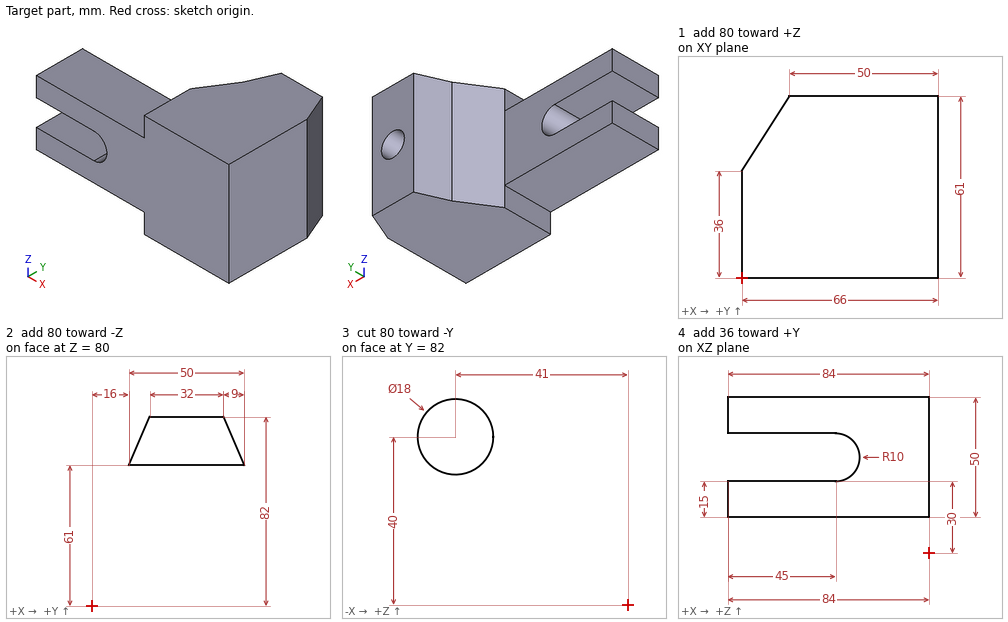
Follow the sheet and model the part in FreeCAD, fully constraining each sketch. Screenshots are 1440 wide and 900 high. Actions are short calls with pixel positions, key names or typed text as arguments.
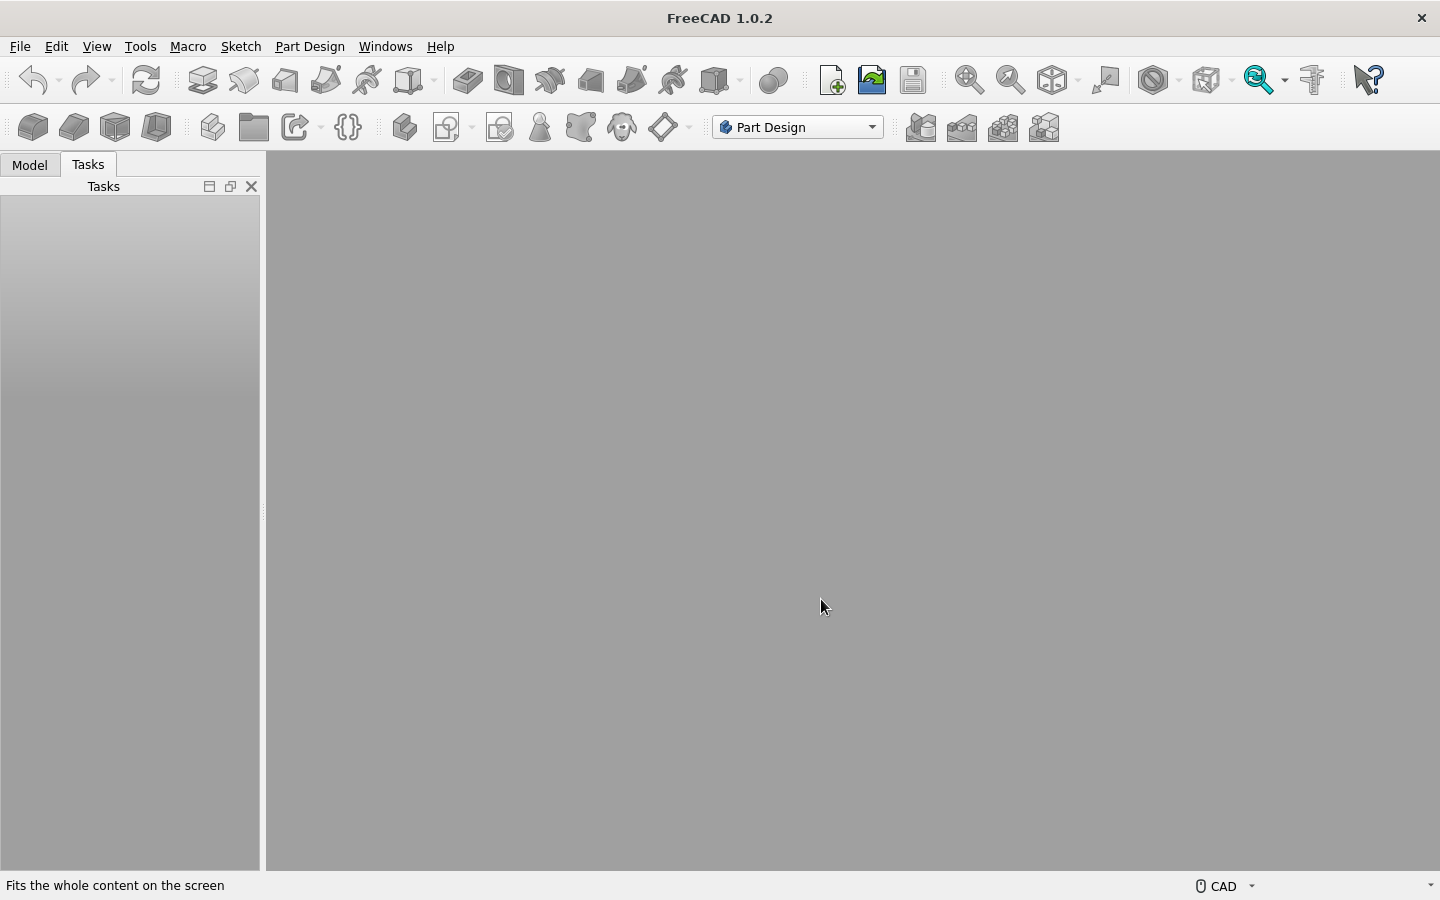
key(ctrl+n)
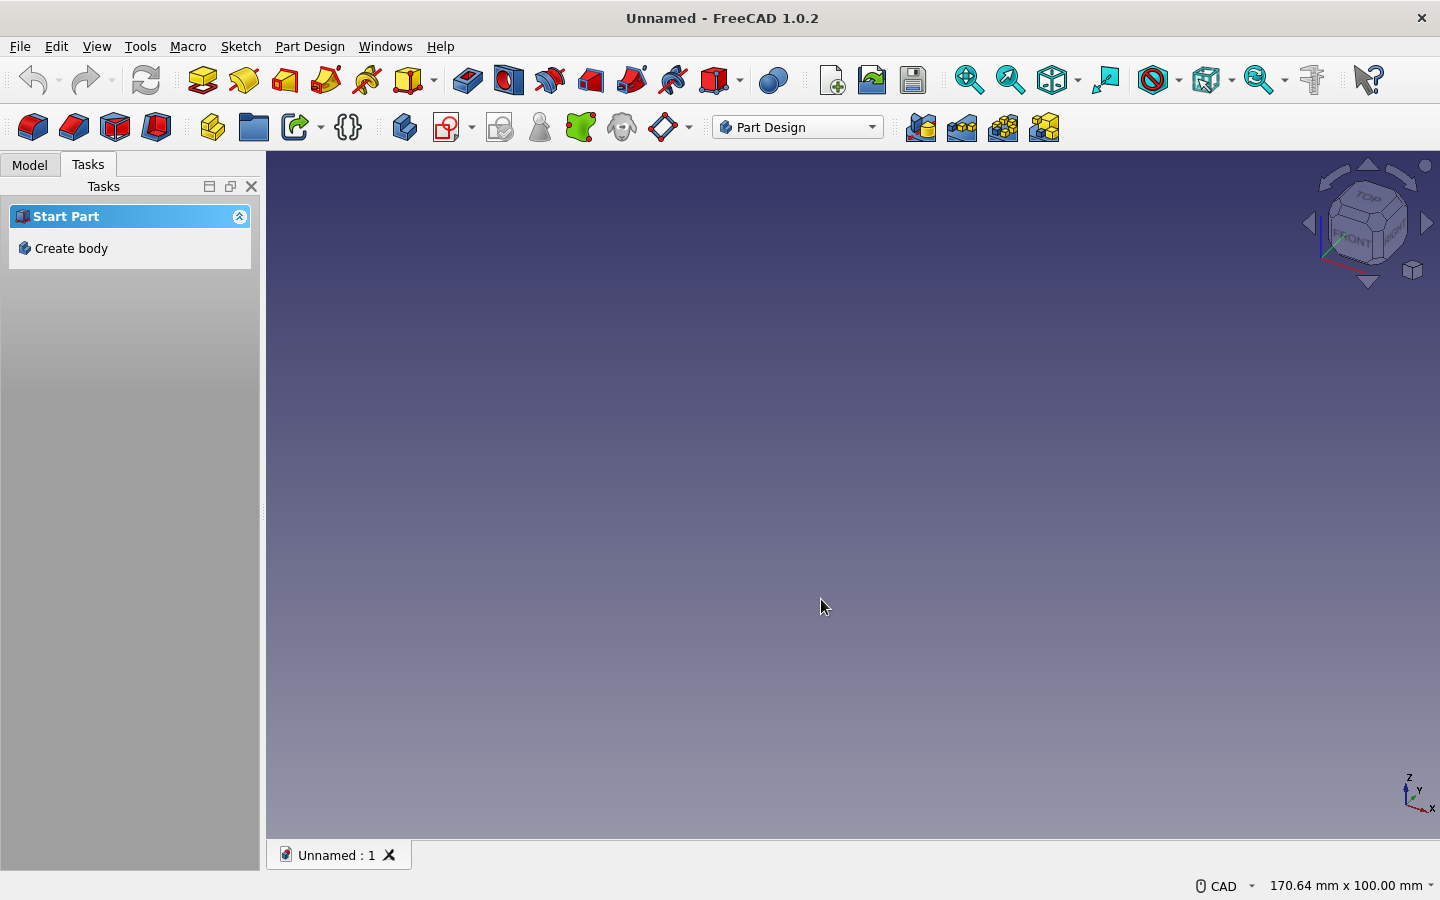
click(446, 128)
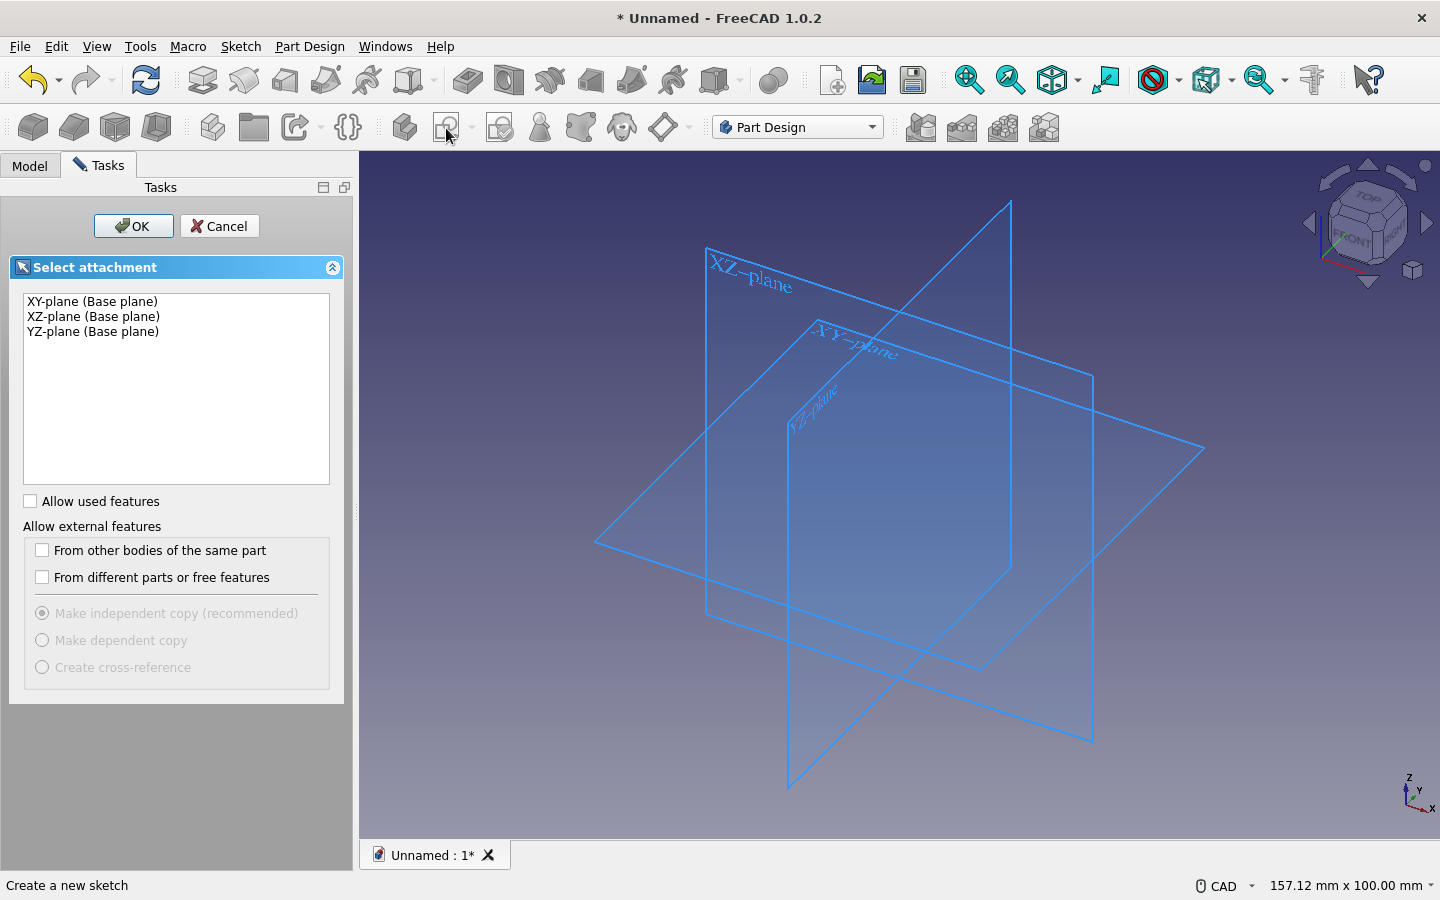
click(84, 302)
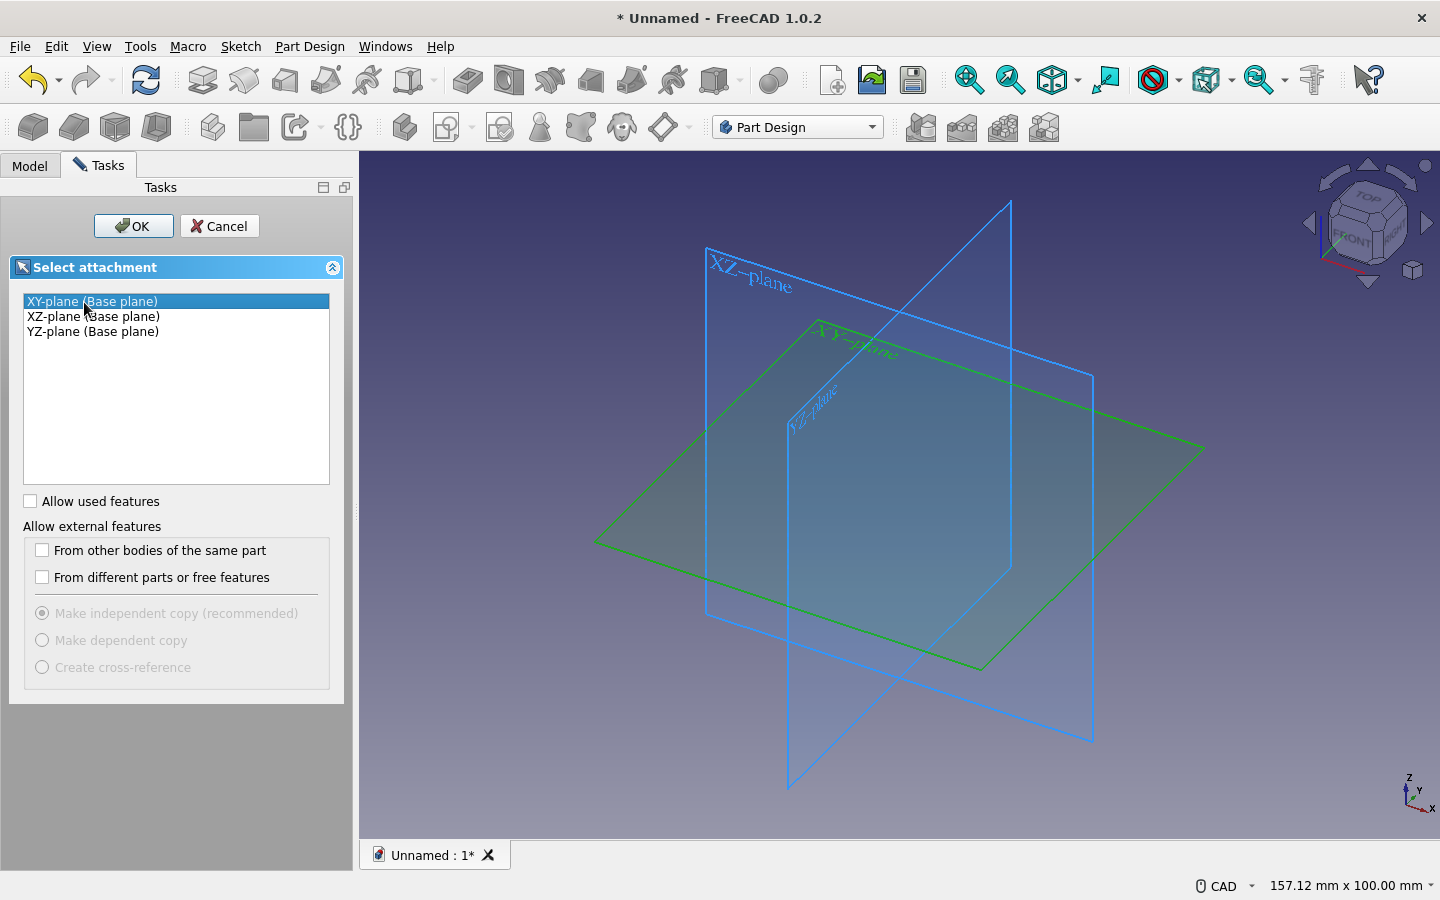
click(134, 226)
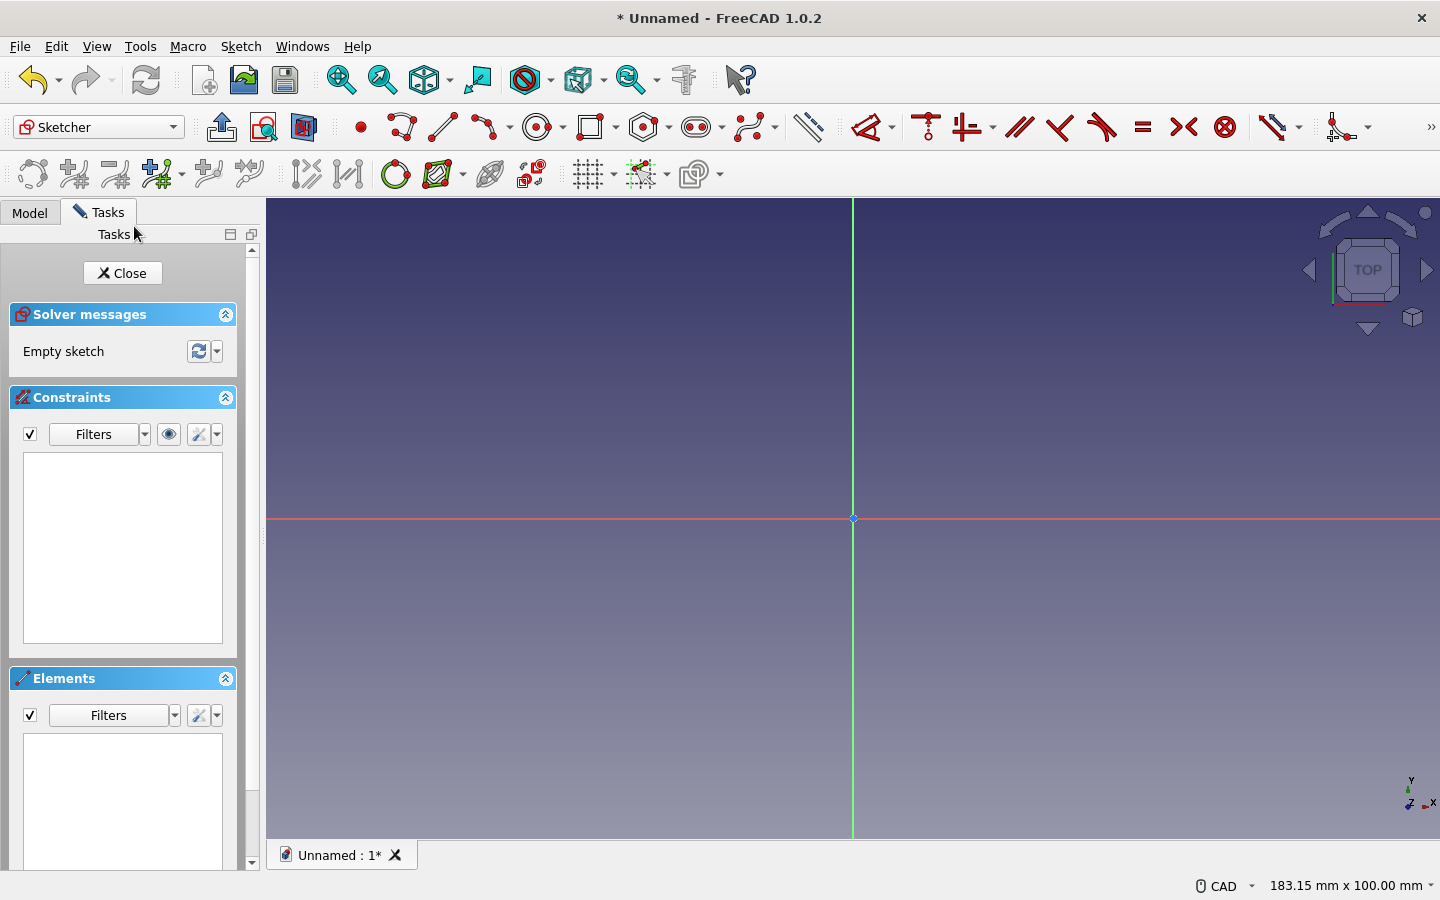
scroll(294, 811, down, 1)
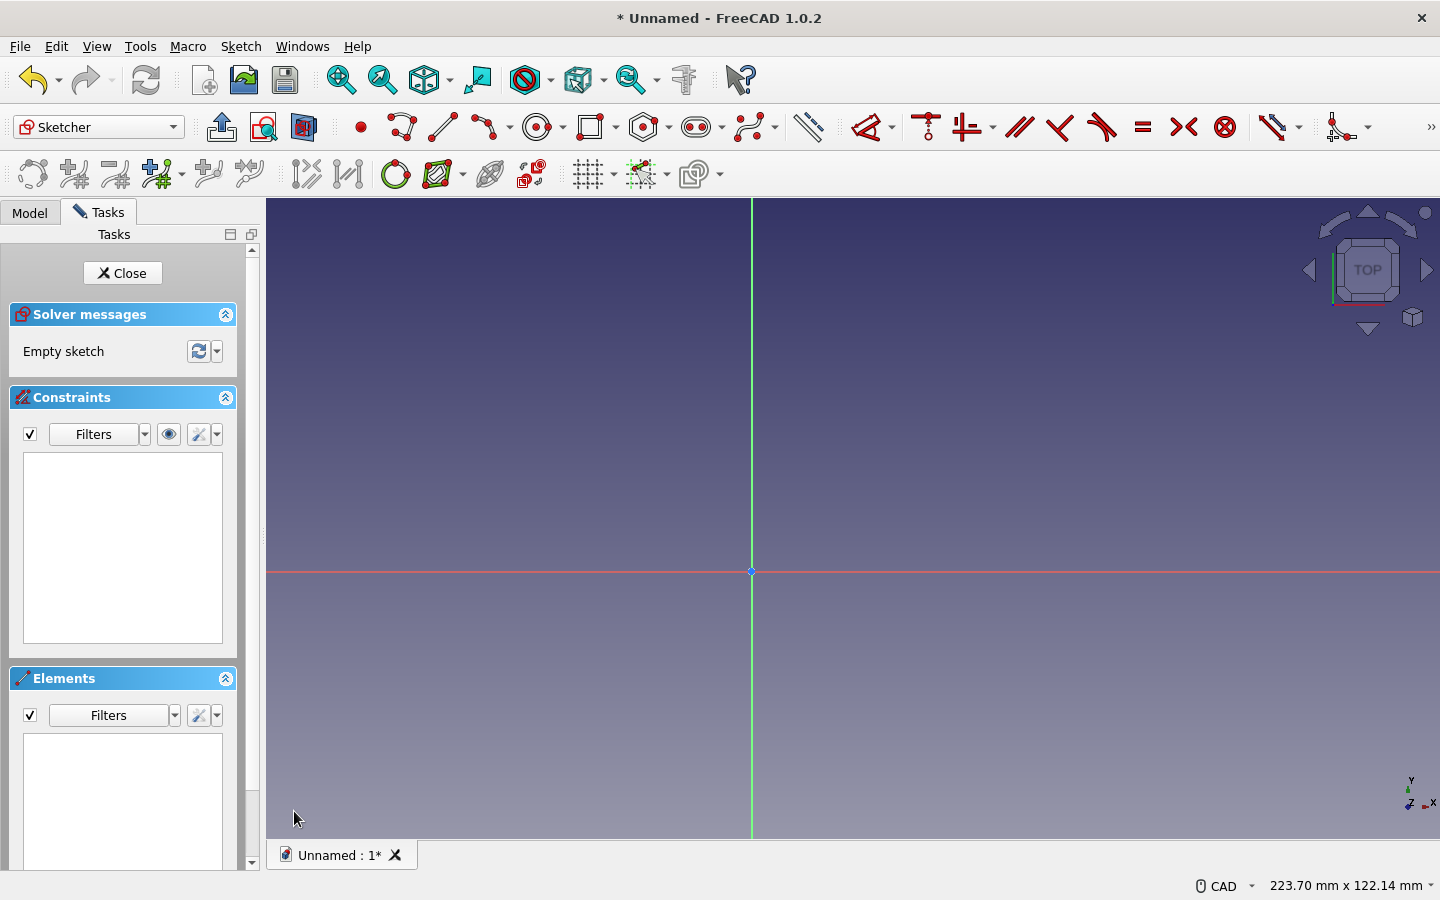
key(g)
key(m)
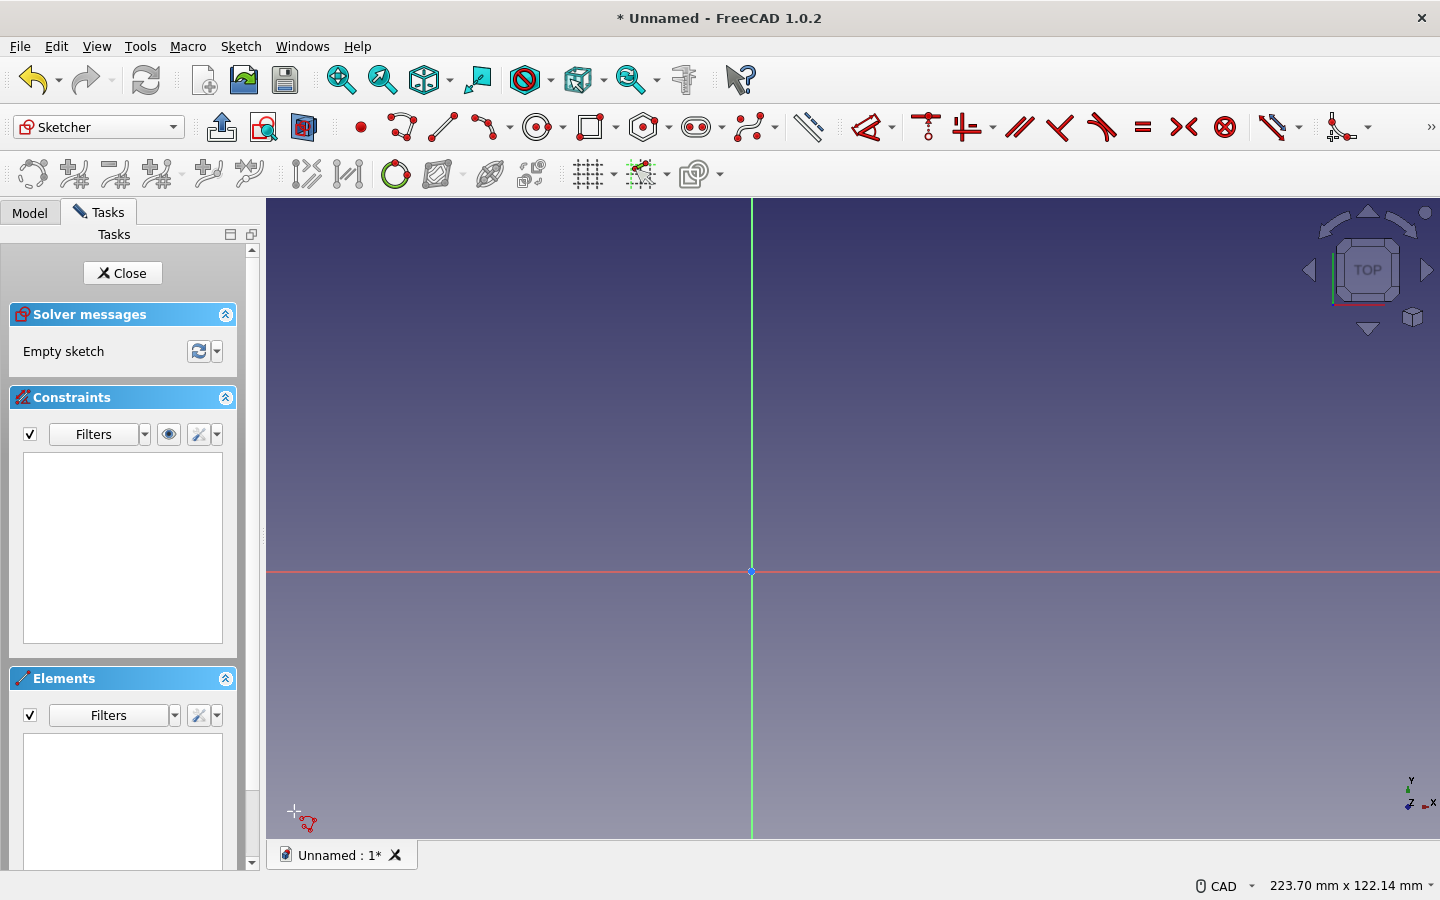
click(752, 572)
click(1098, 563)
click(1098, 252)
click(836, 252)
click(761, 383)
click(752, 572)
key(Escape)
key(Escape)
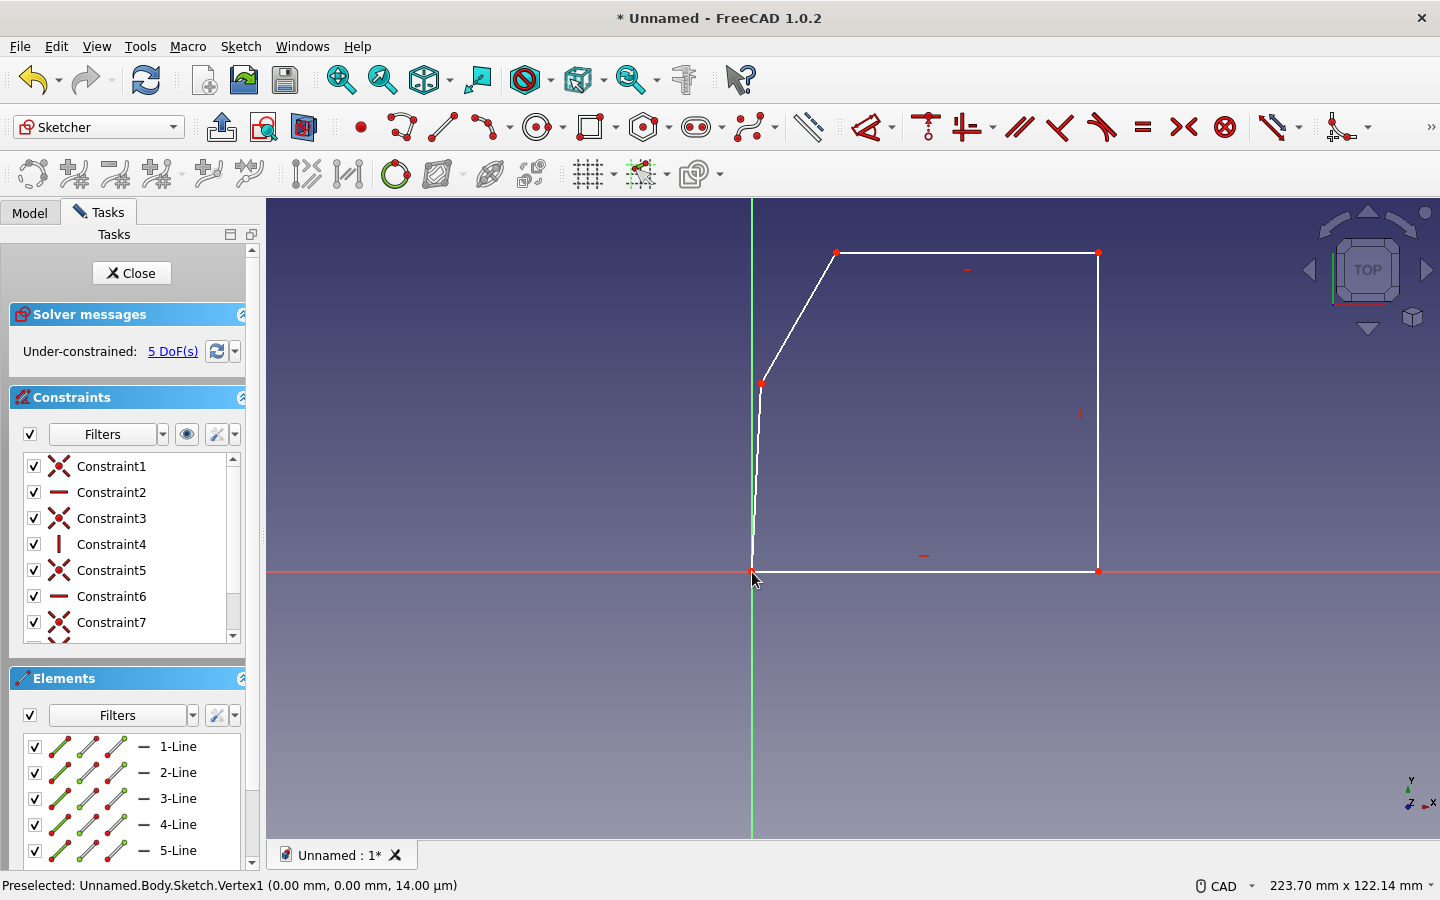
click(754, 515)